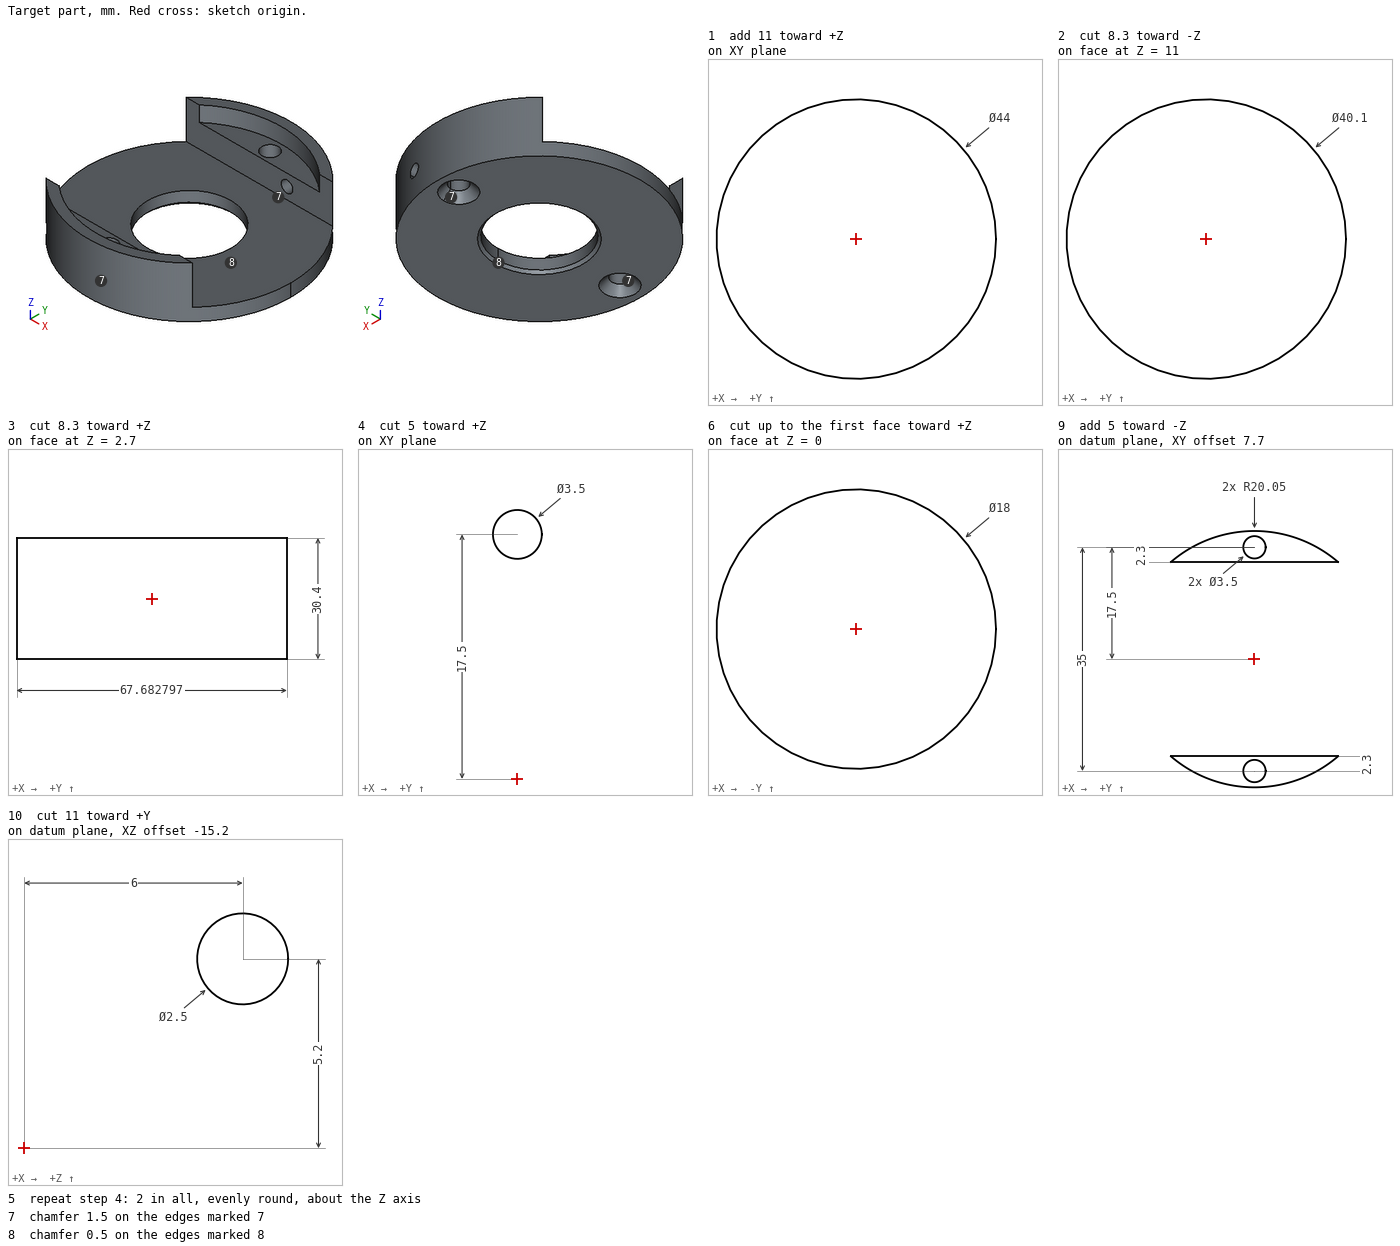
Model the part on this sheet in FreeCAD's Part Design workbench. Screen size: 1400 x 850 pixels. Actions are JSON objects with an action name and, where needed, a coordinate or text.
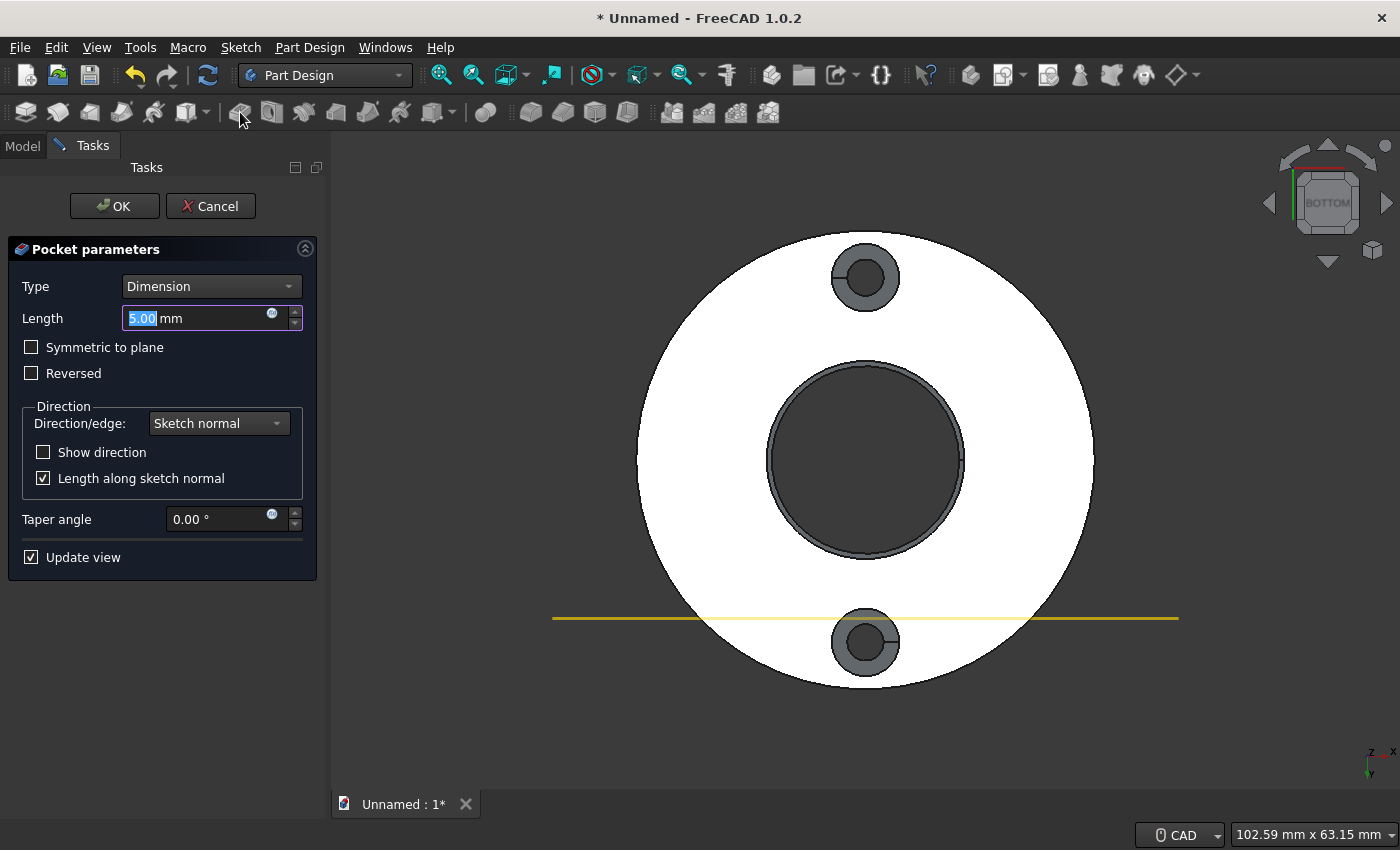
{"action": "type", "text": "11"}
{"action": "key", "text": "Tab"}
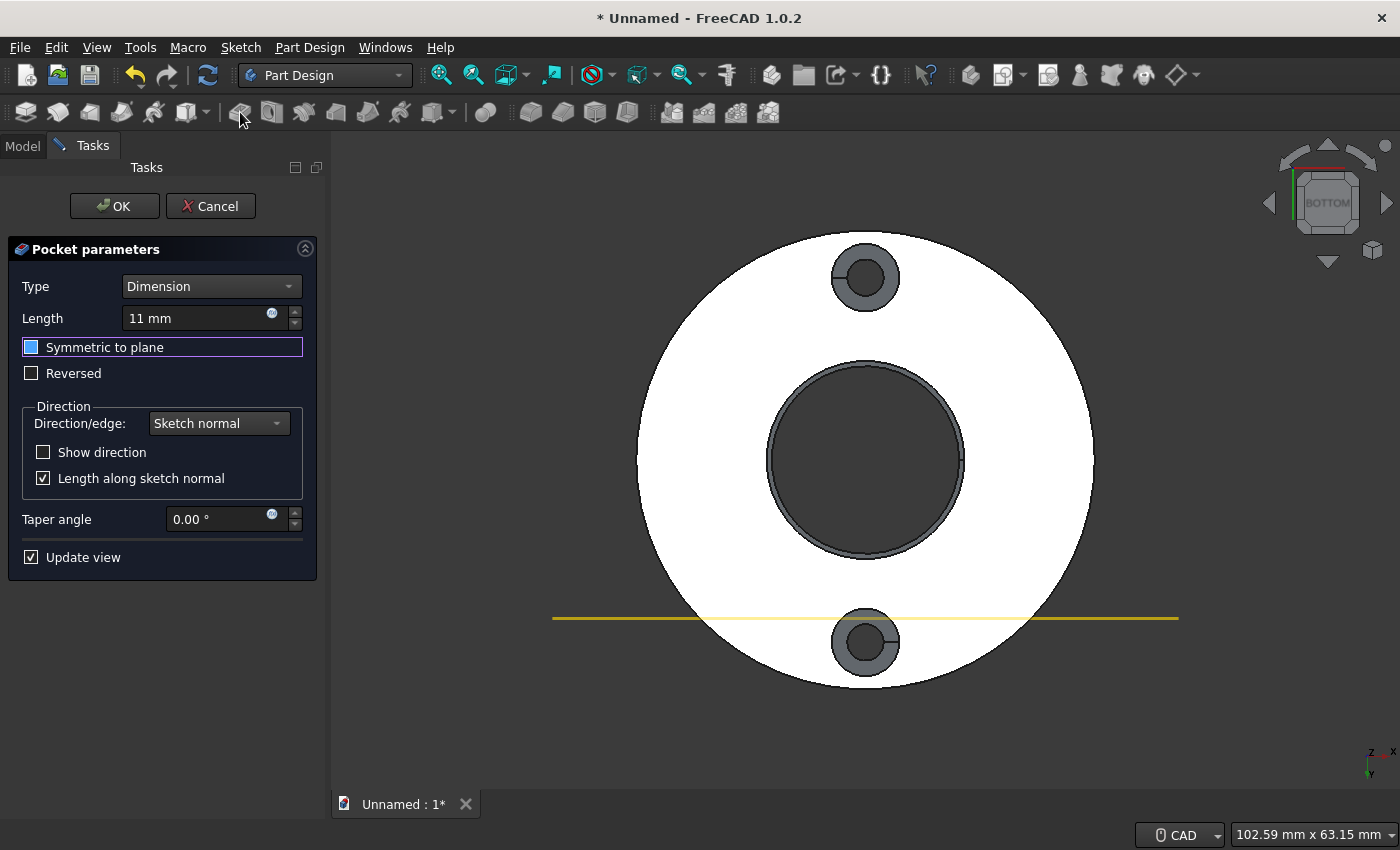
{"action": "left_click", "coordinate": [115, 206]}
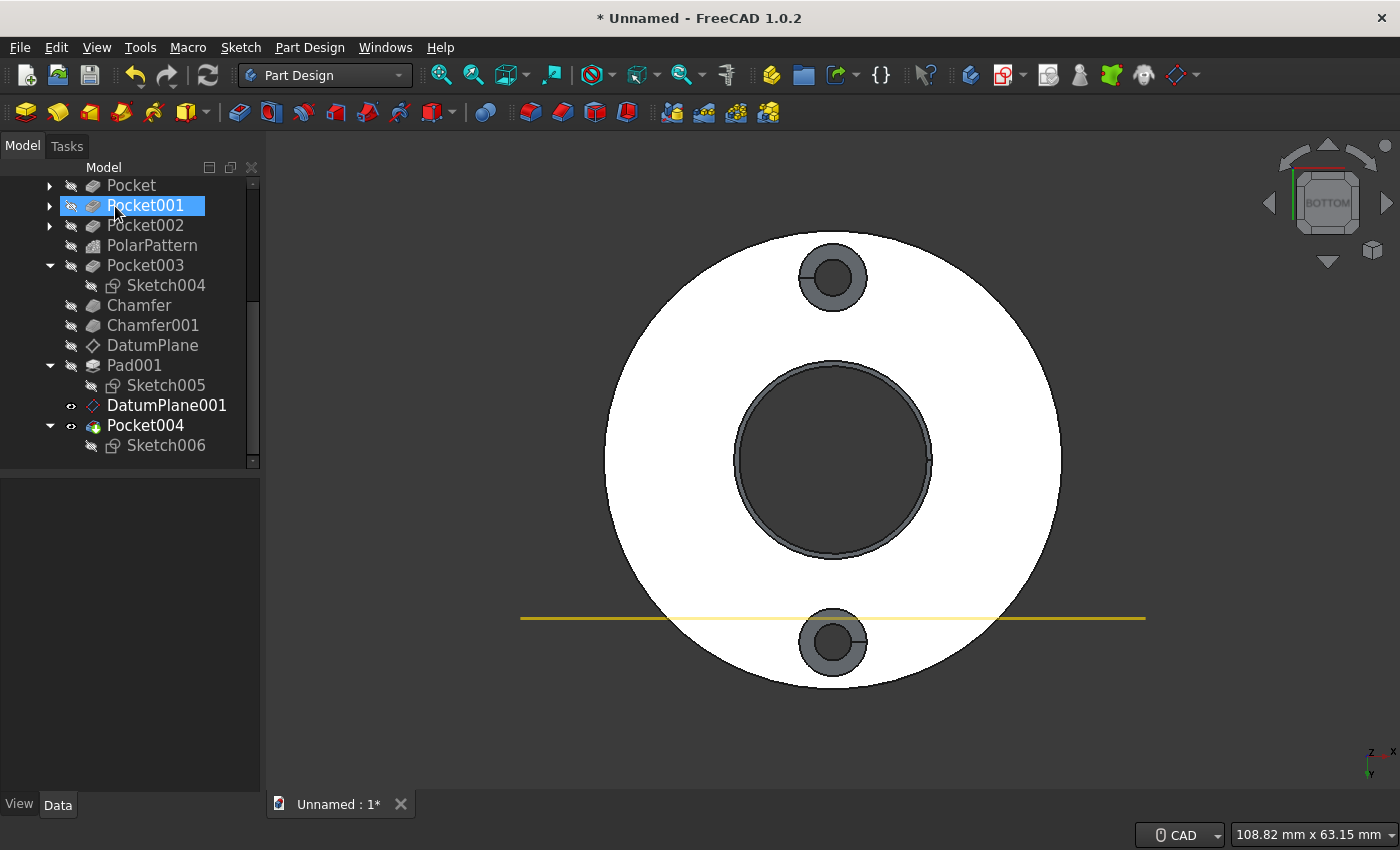
{"action": "left_click", "coordinate": [116, 406]}
{"action": "key", "text": "space"}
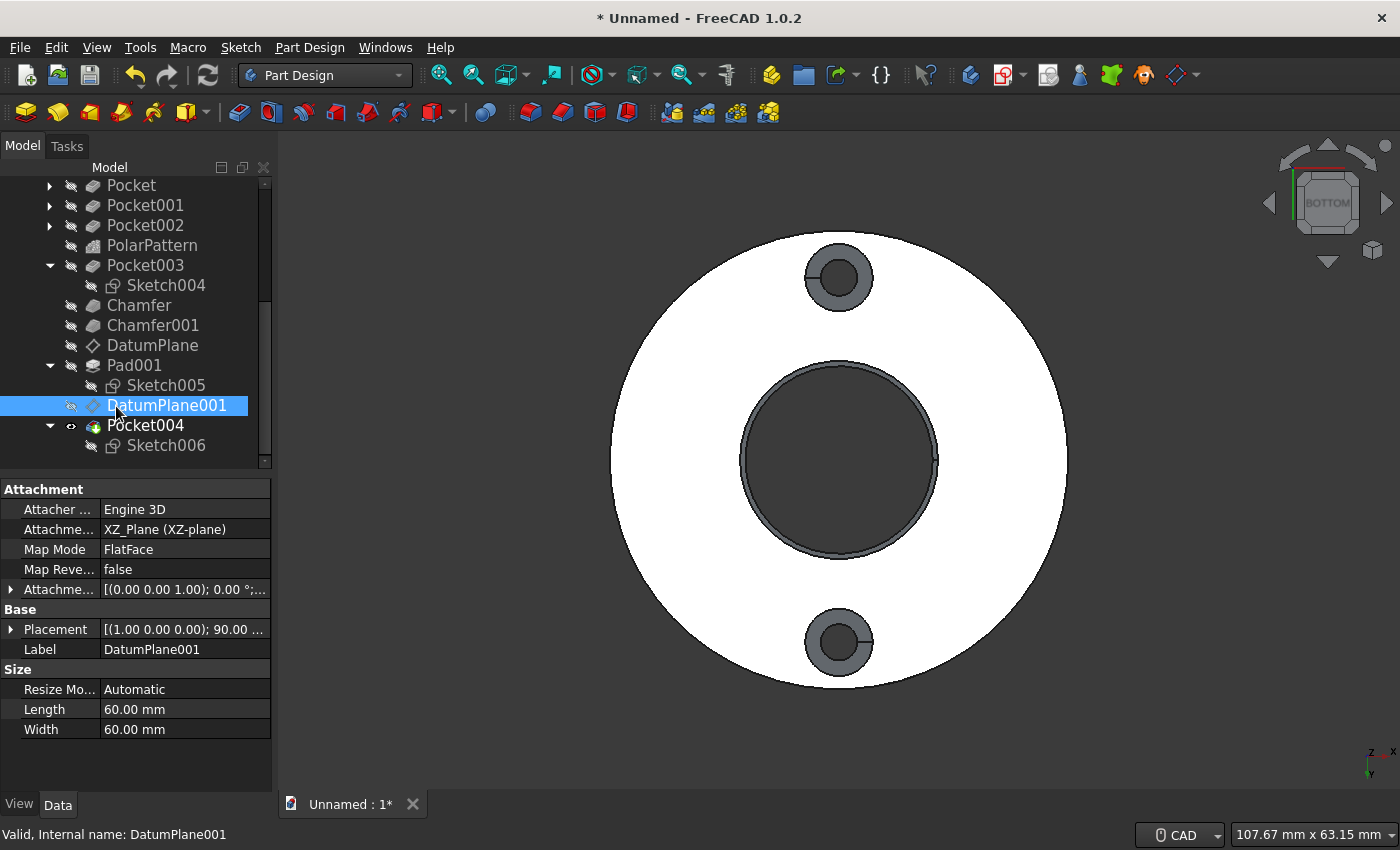
{"action": "key", "text": "0"}